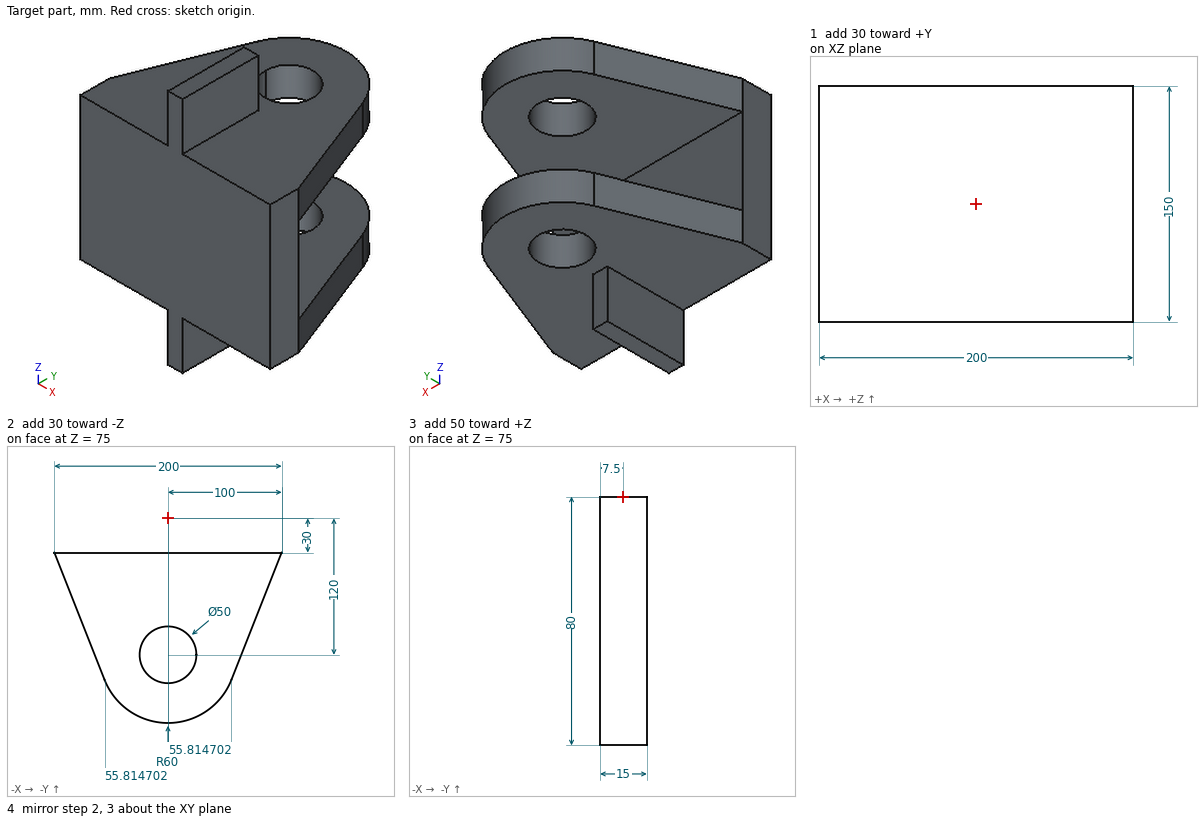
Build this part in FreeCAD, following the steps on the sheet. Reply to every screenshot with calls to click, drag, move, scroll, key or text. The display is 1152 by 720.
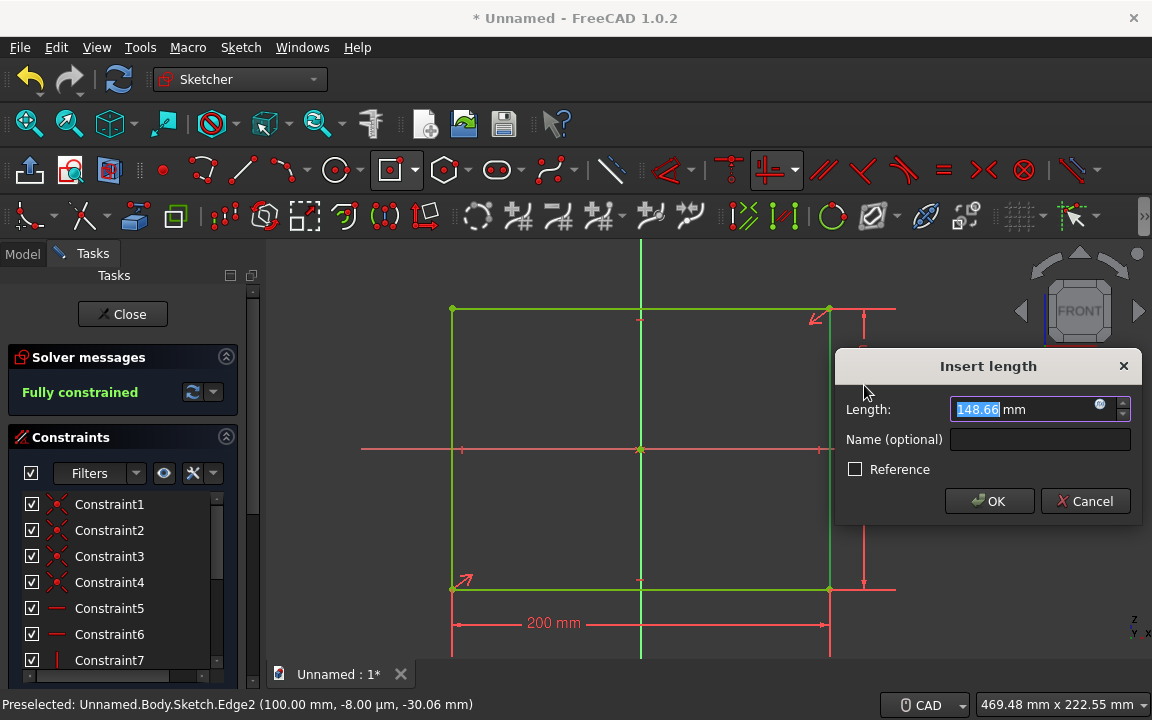
text(150)
key(Return)
key(Escape)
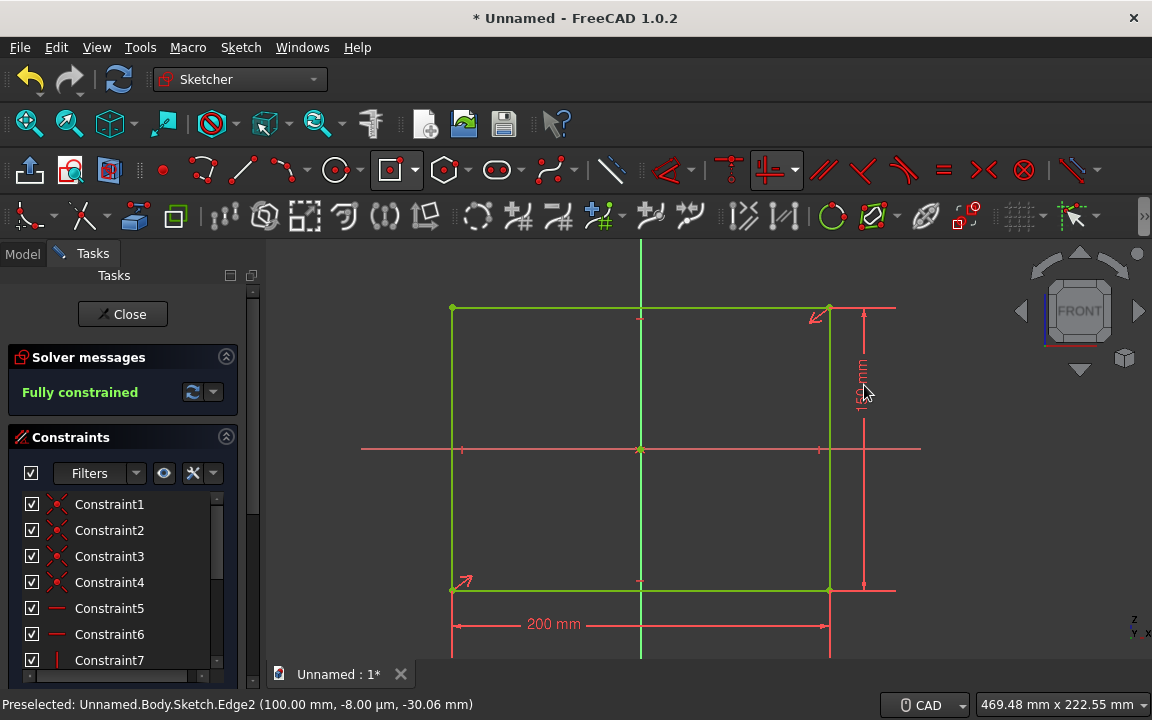
click(123, 314)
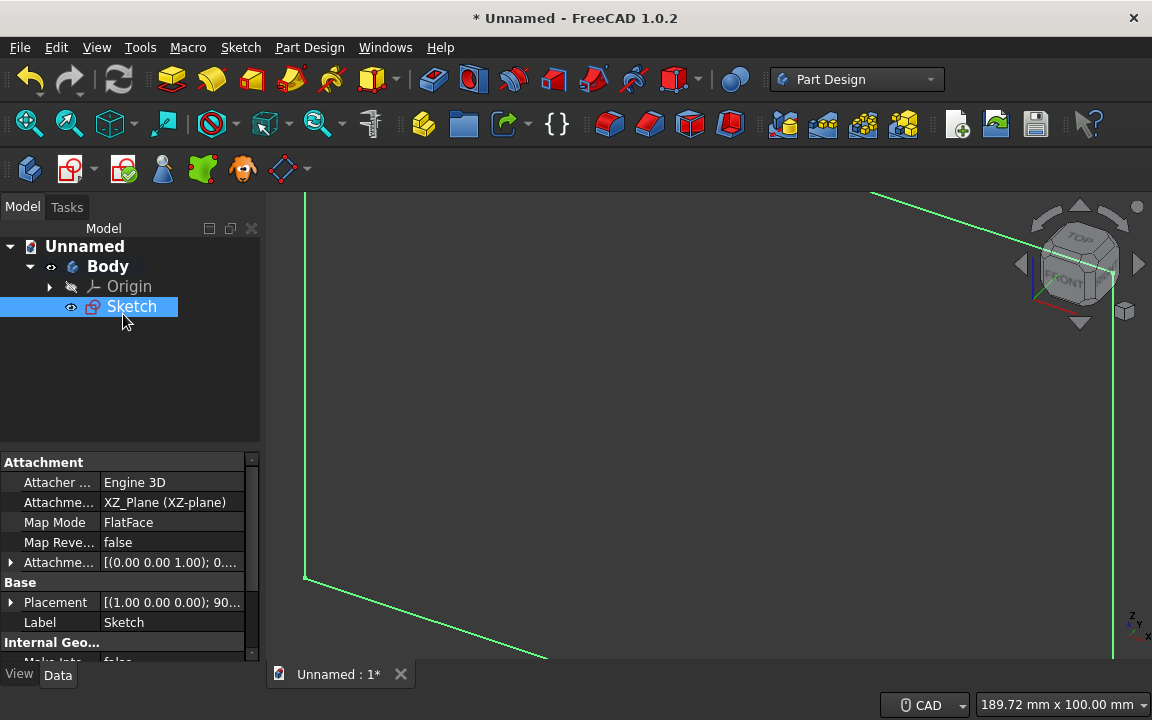
click(172, 80)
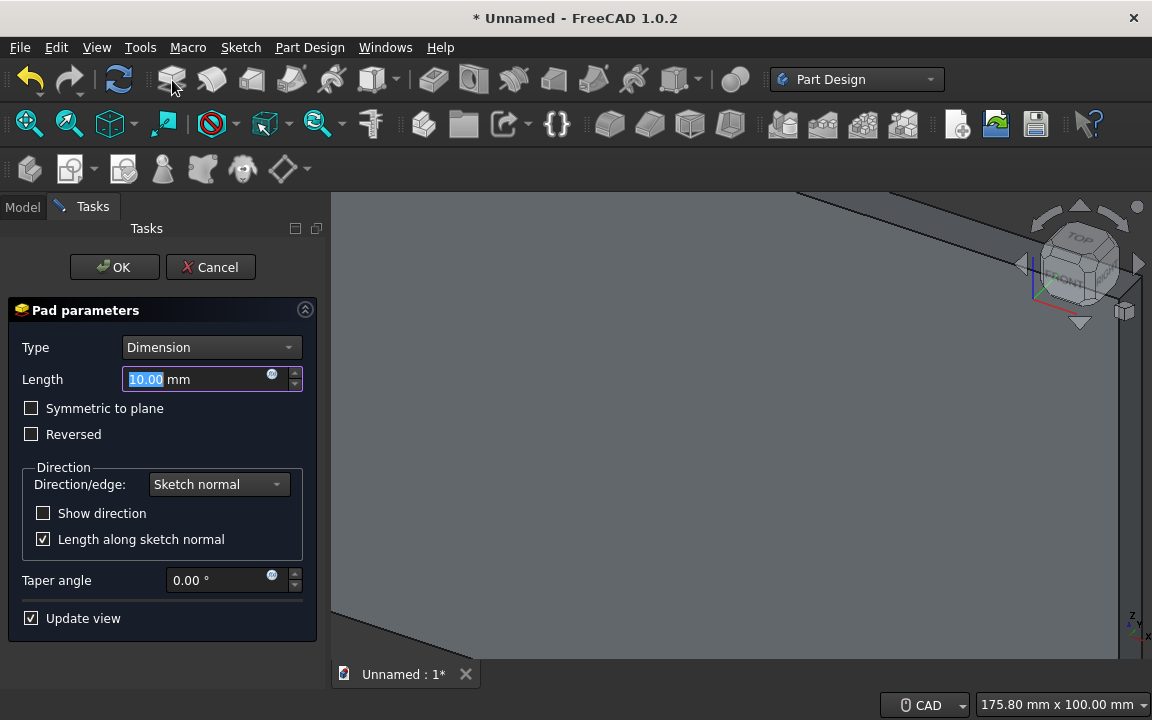
text(30)
key(Tab)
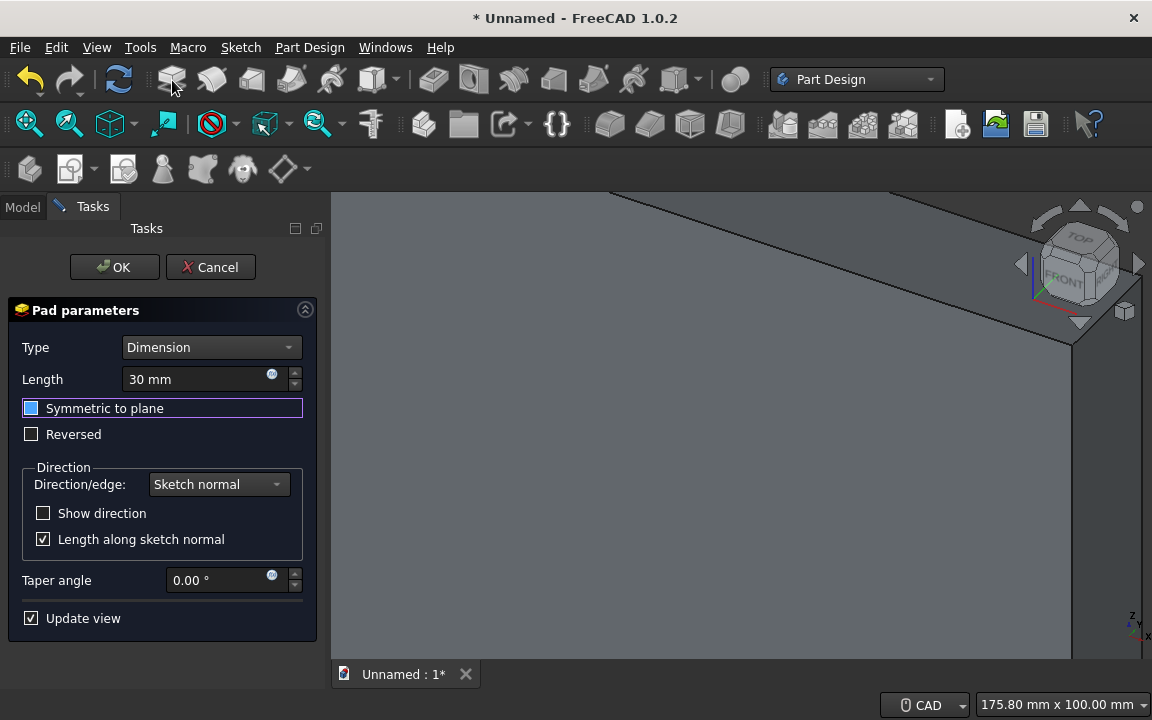
click(30, 434)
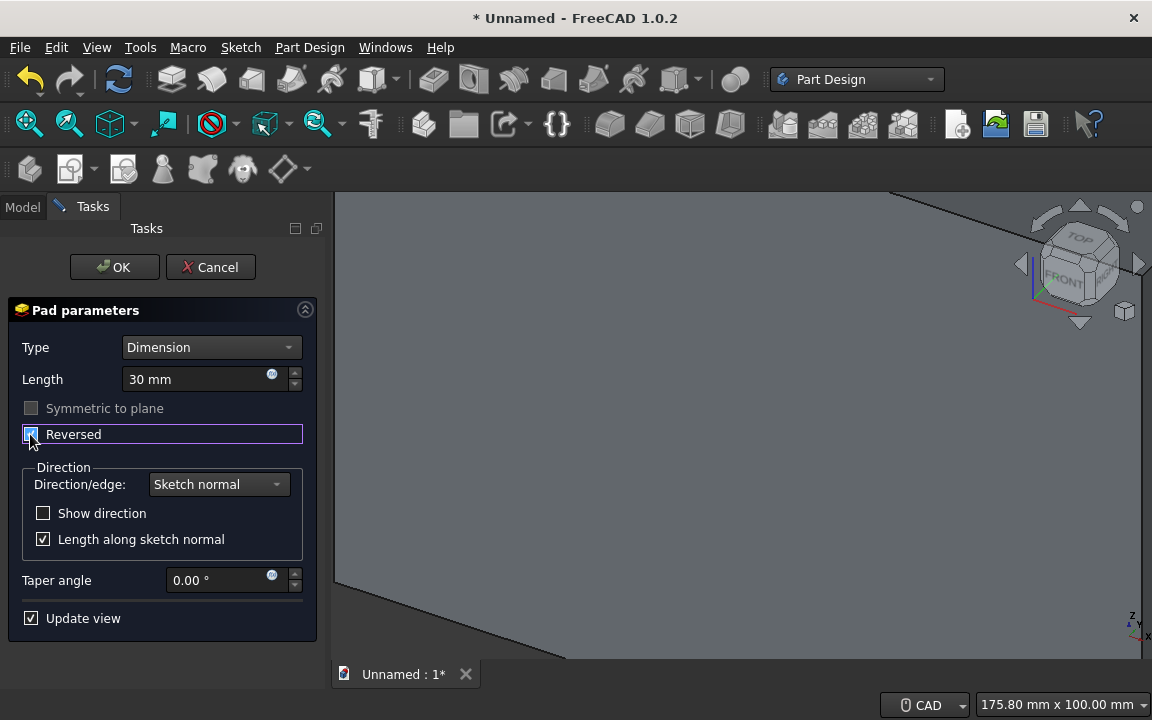
click(115, 267)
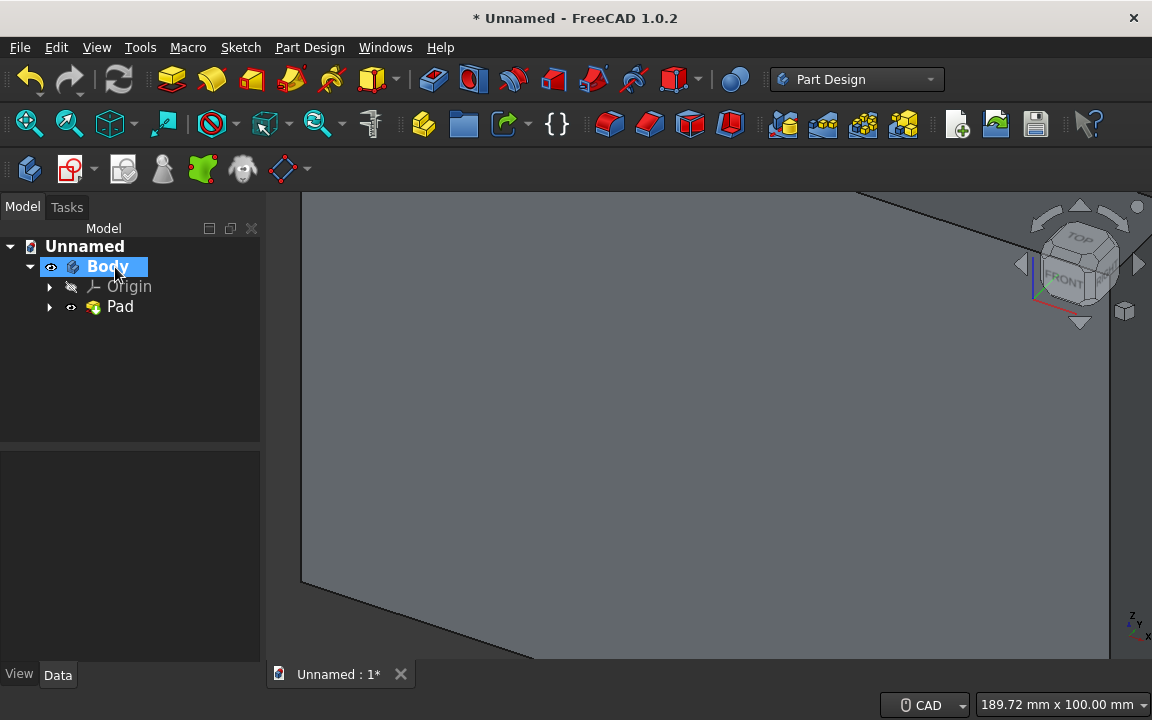
key(v)
key(f)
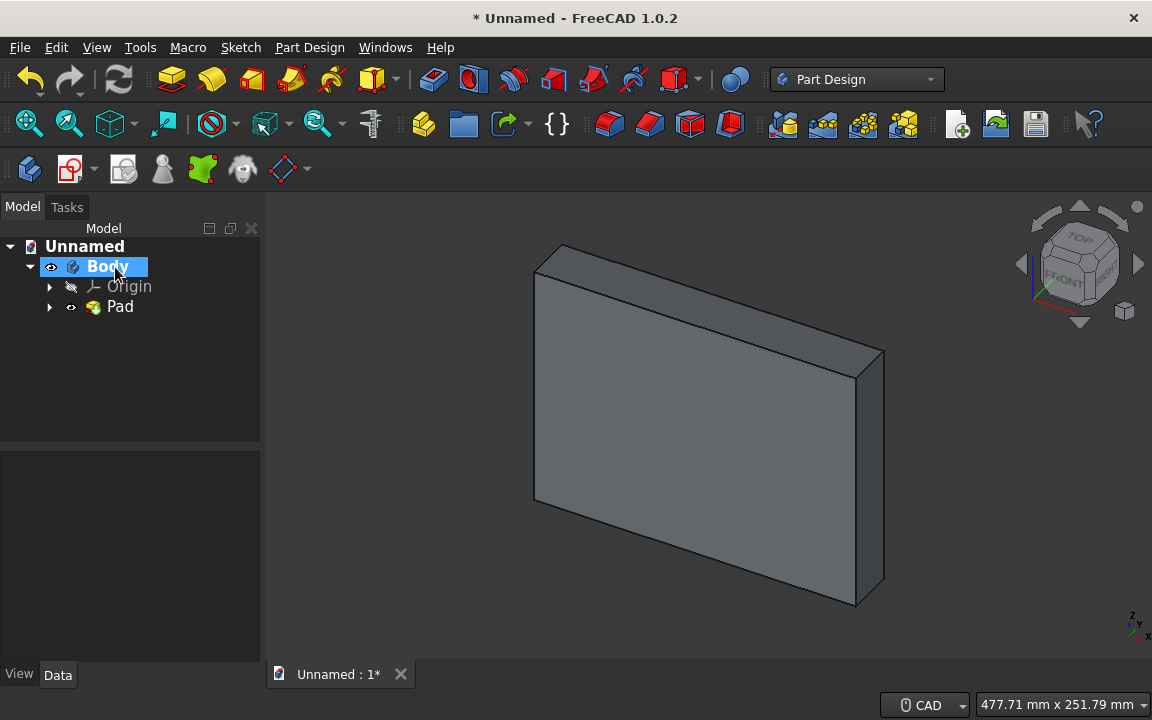
click(801, 341)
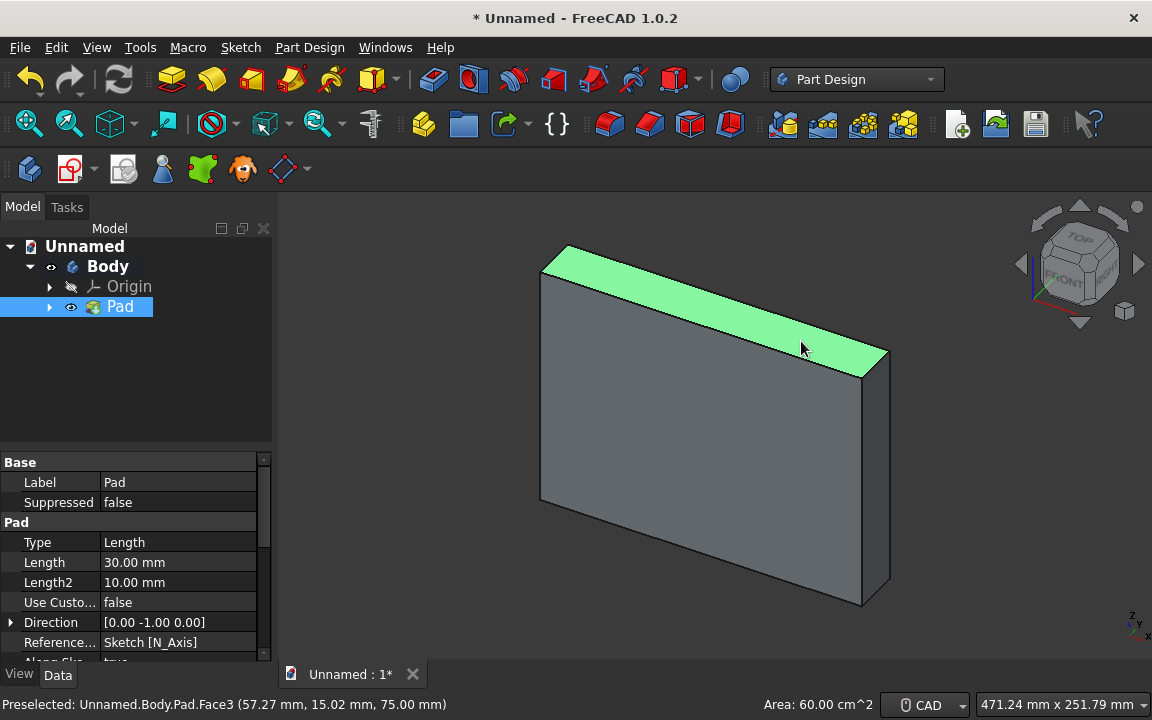
click(70, 170)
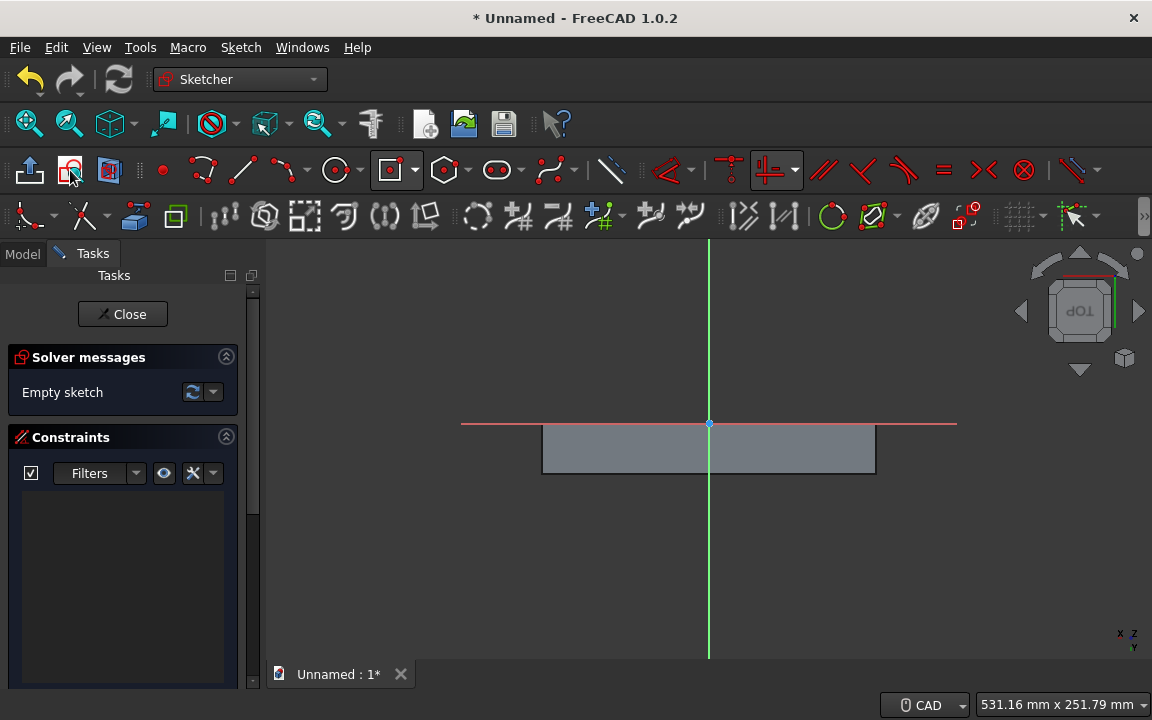
scroll(501, 267, down, 2)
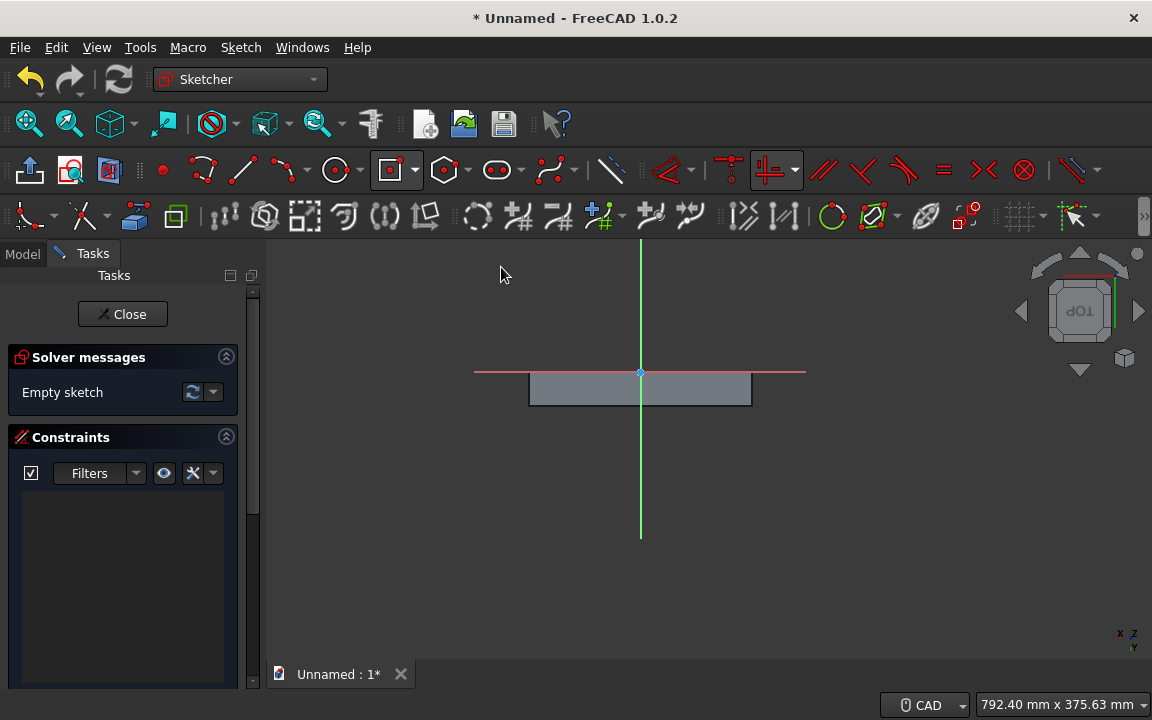
key(g)
key(m)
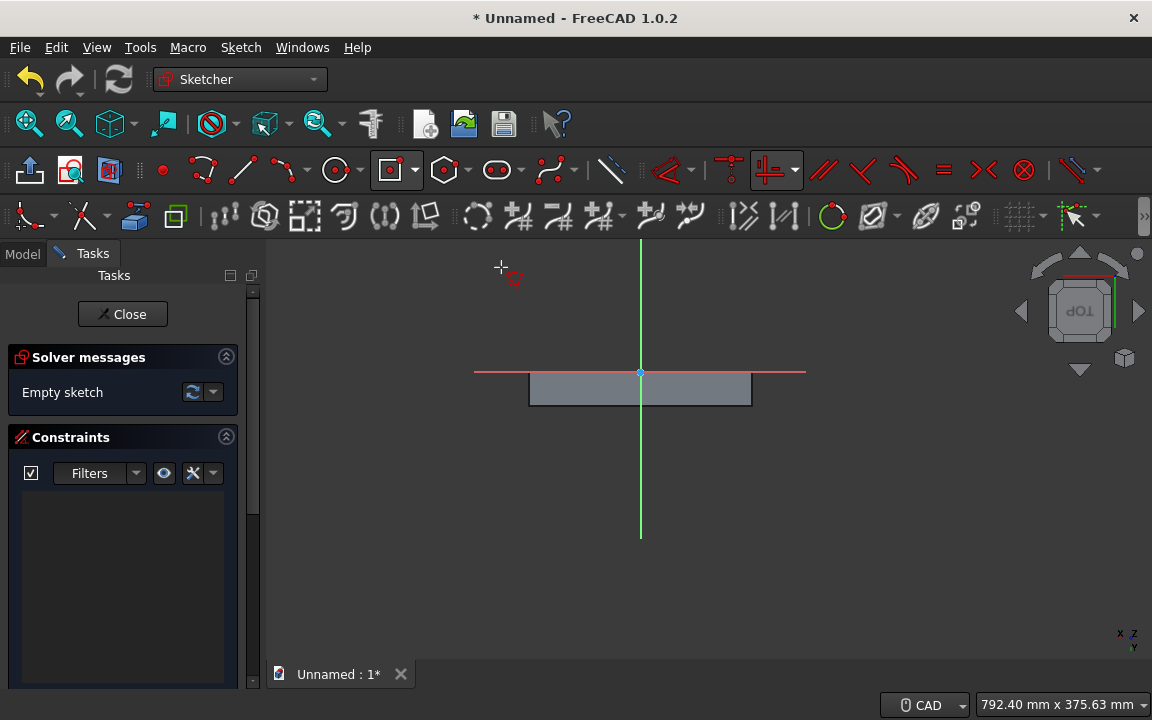
click(703, 531)
click(752, 406)
click(529, 406)
click(578, 531)
right_click(578, 531)